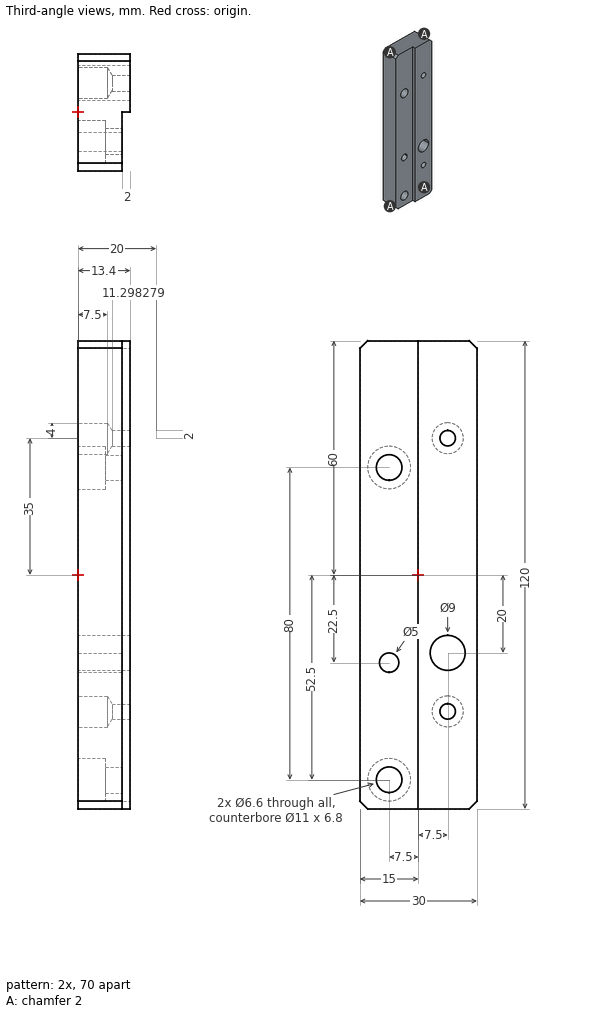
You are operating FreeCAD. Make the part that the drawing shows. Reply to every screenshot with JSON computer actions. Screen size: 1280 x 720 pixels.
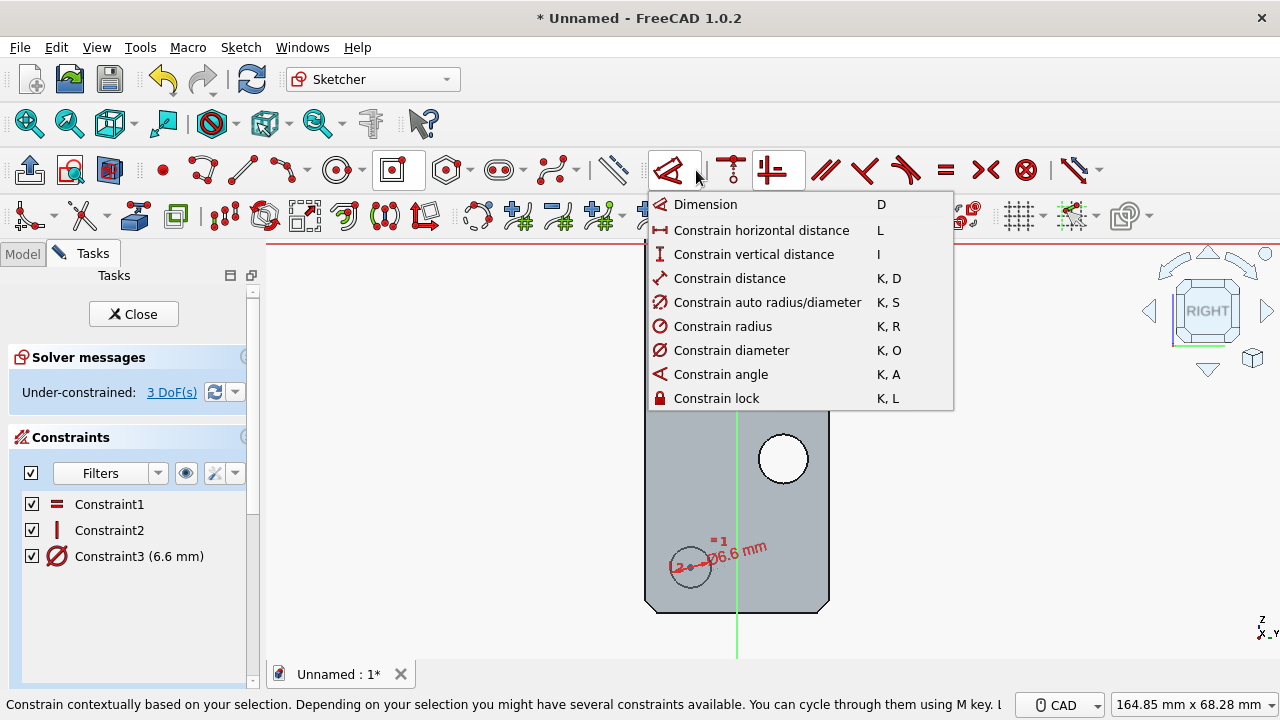
{"action": "left_click", "coordinate": [801, 230]}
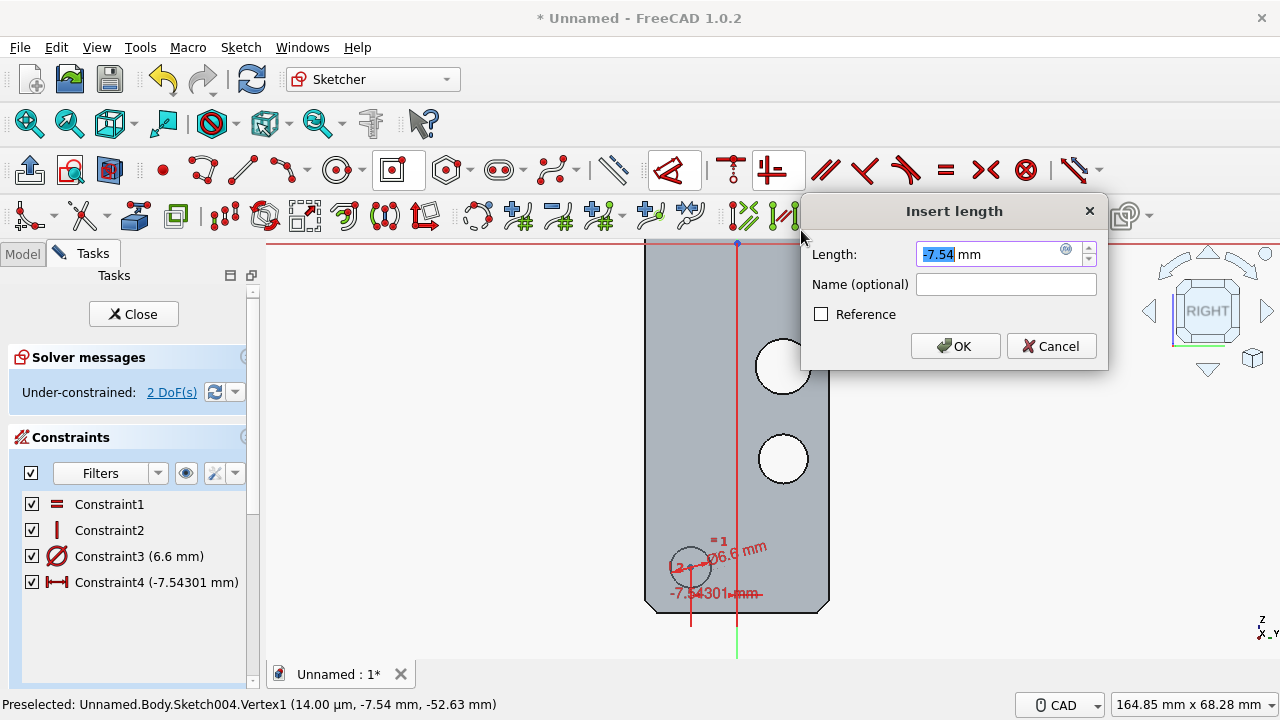
{"action": "type", "text": "-7.5"}
{"action": "key", "text": "Return"}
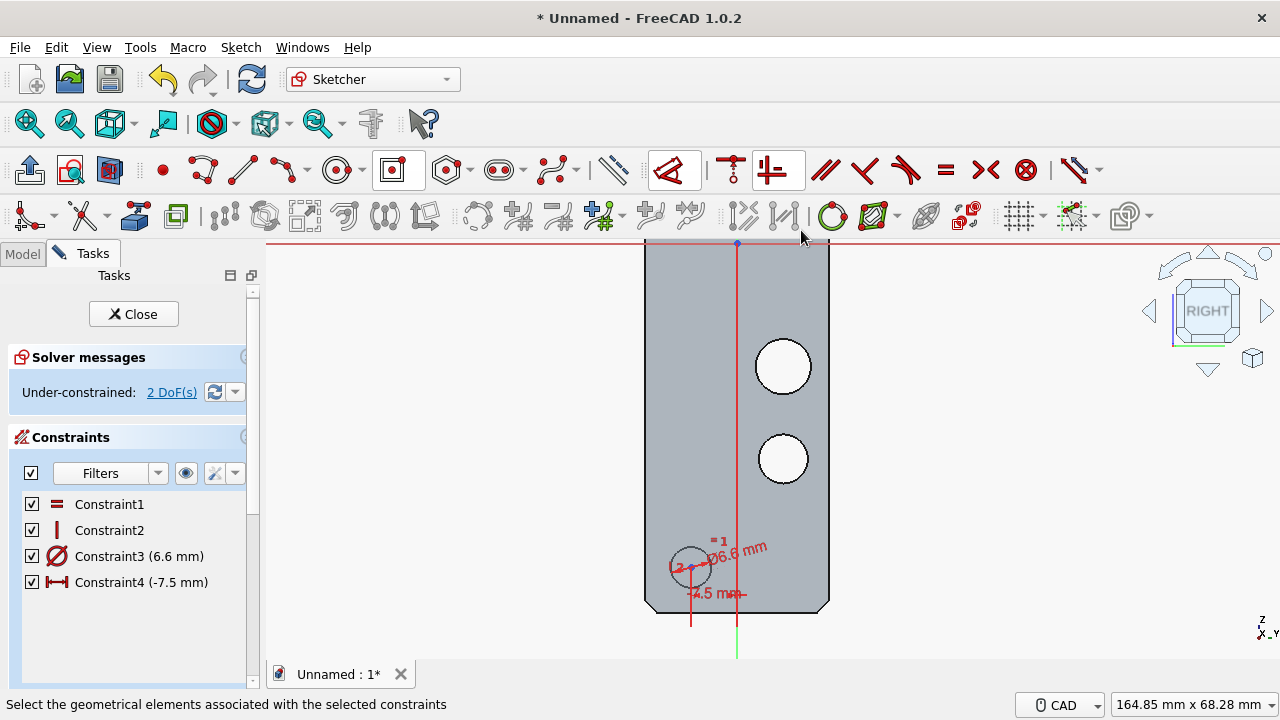
{"action": "left_click", "coordinate": [691, 567]}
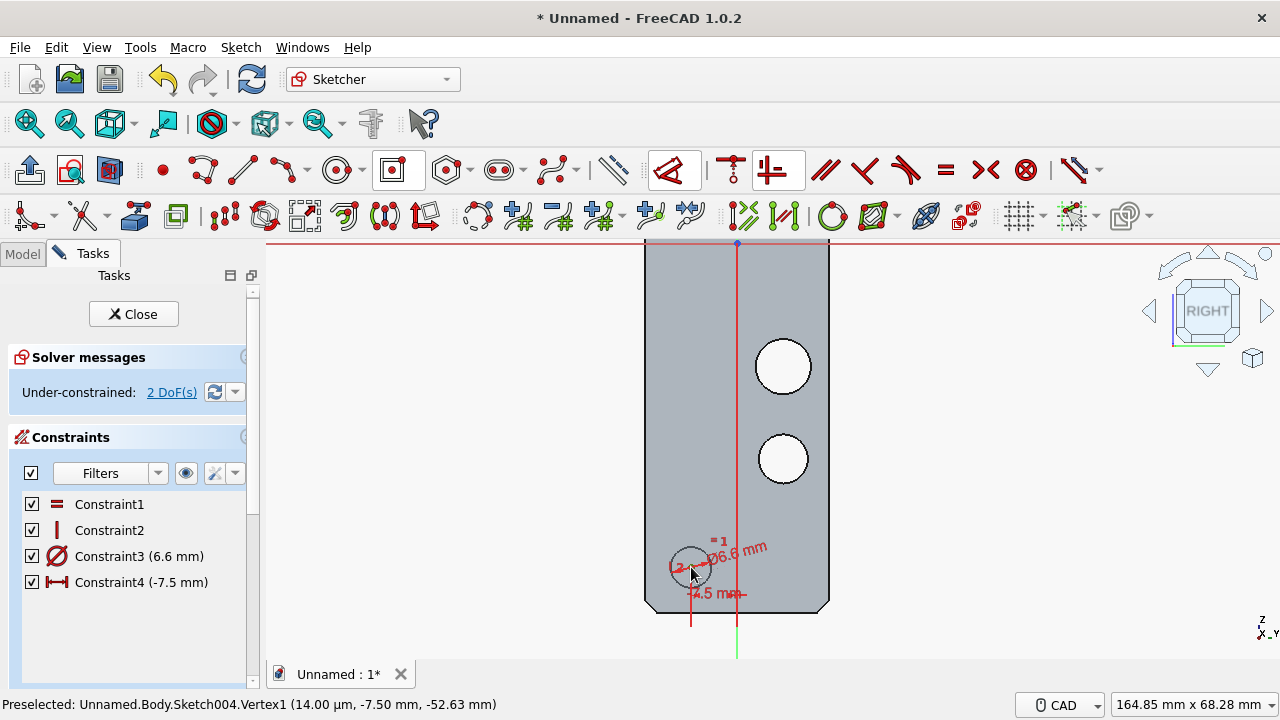
{"action": "scroll", "coordinate": [705, 554], "scroll_direction": "down", "scroll_amount": 4}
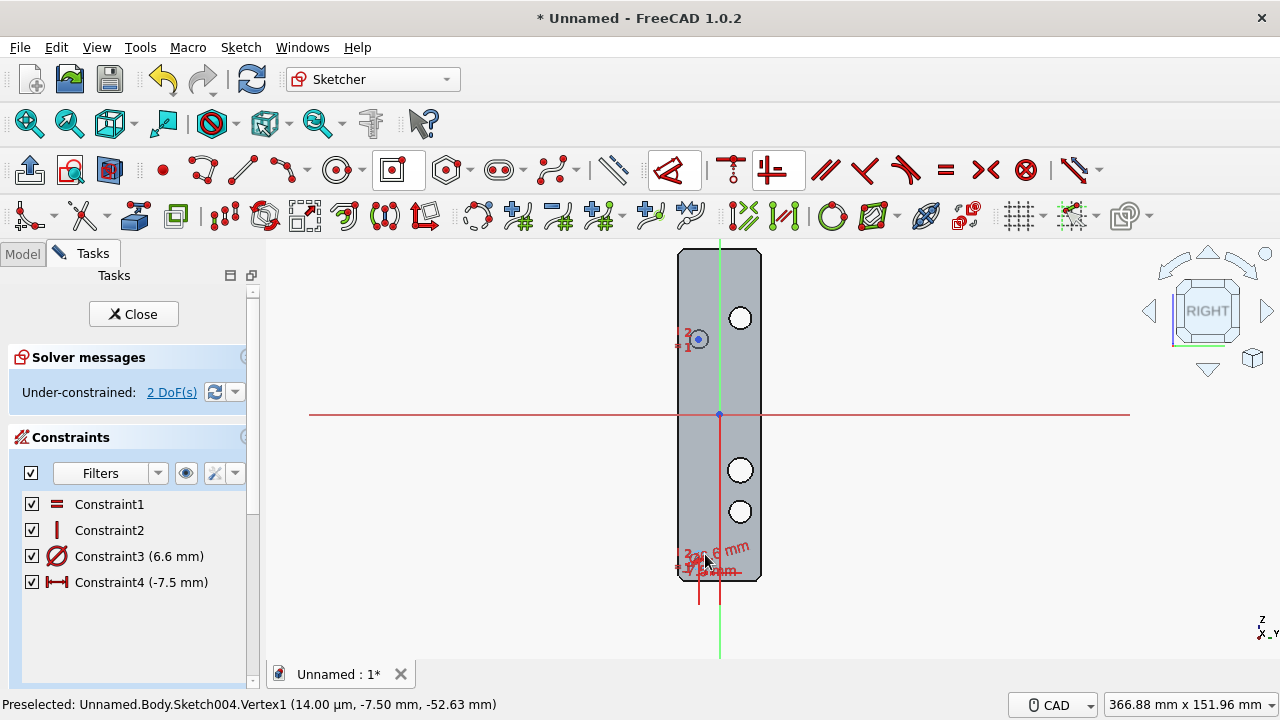
{"action": "left_click", "coordinate": [699, 339]}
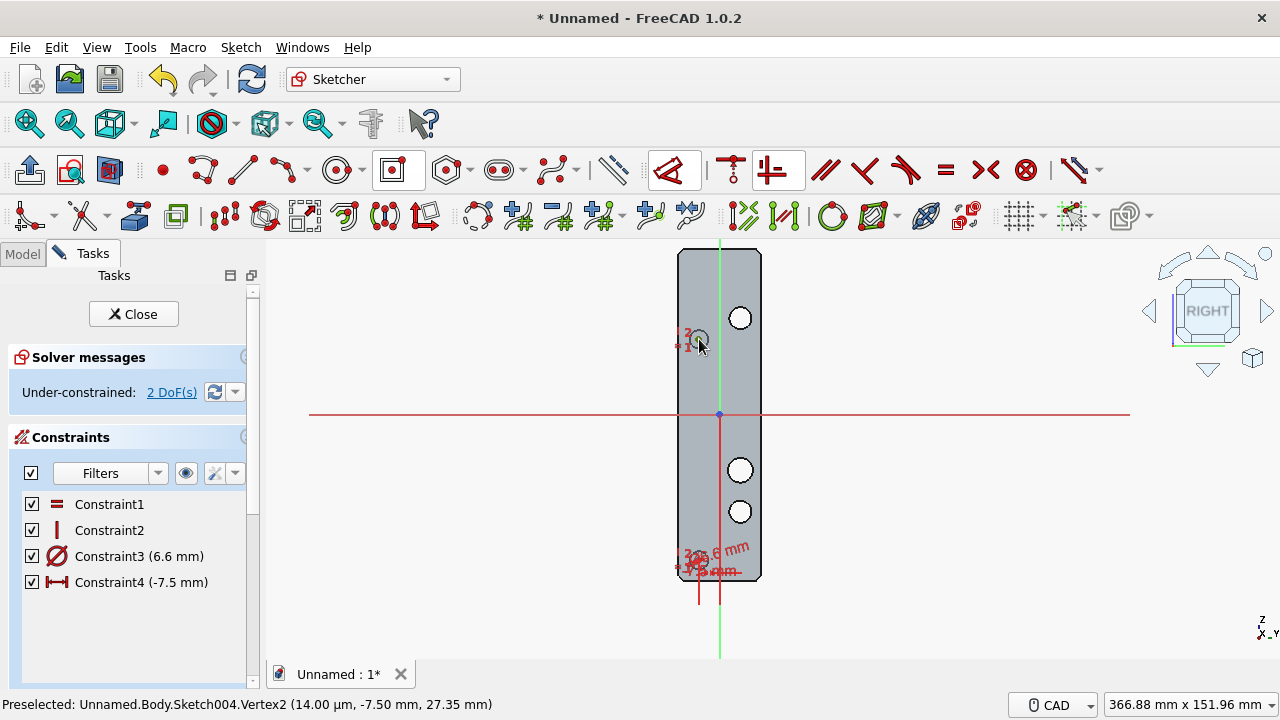
{"action": "key", "text": "i"}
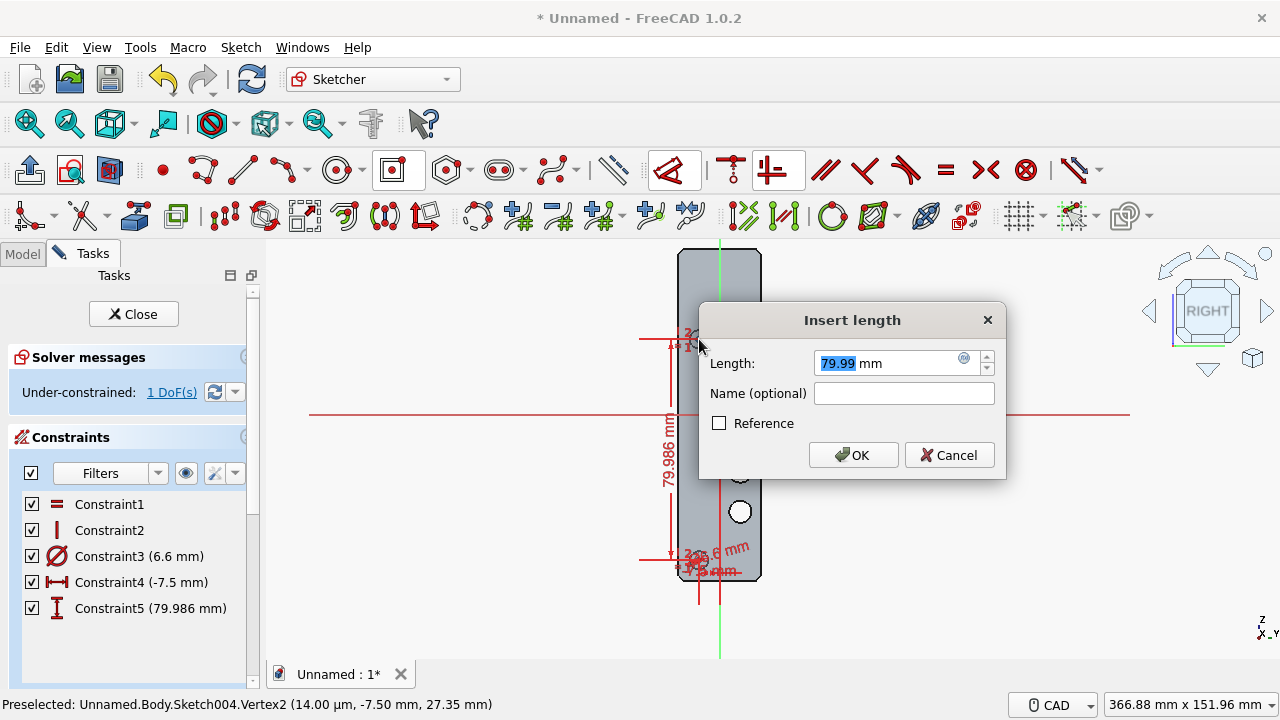
{"action": "type", "text": "80"}
{"action": "key", "text": "Return"}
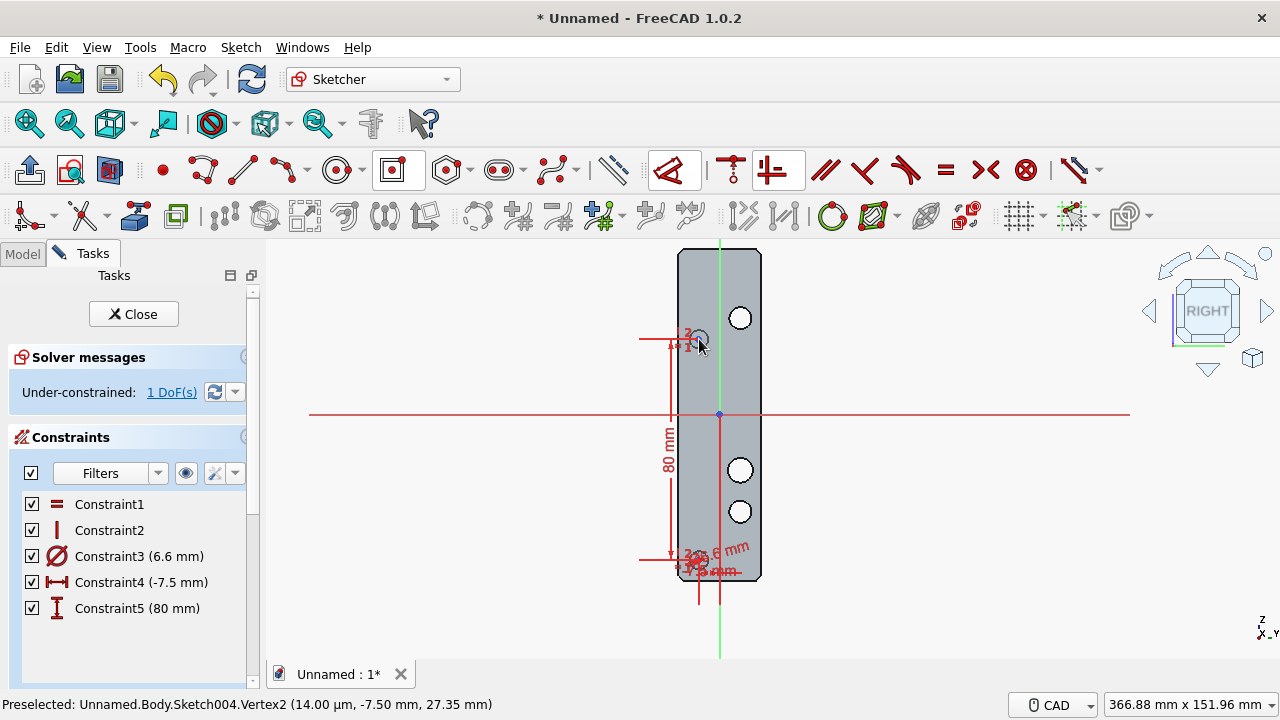
{"action": "left_click", "coordinate": [699, 560]}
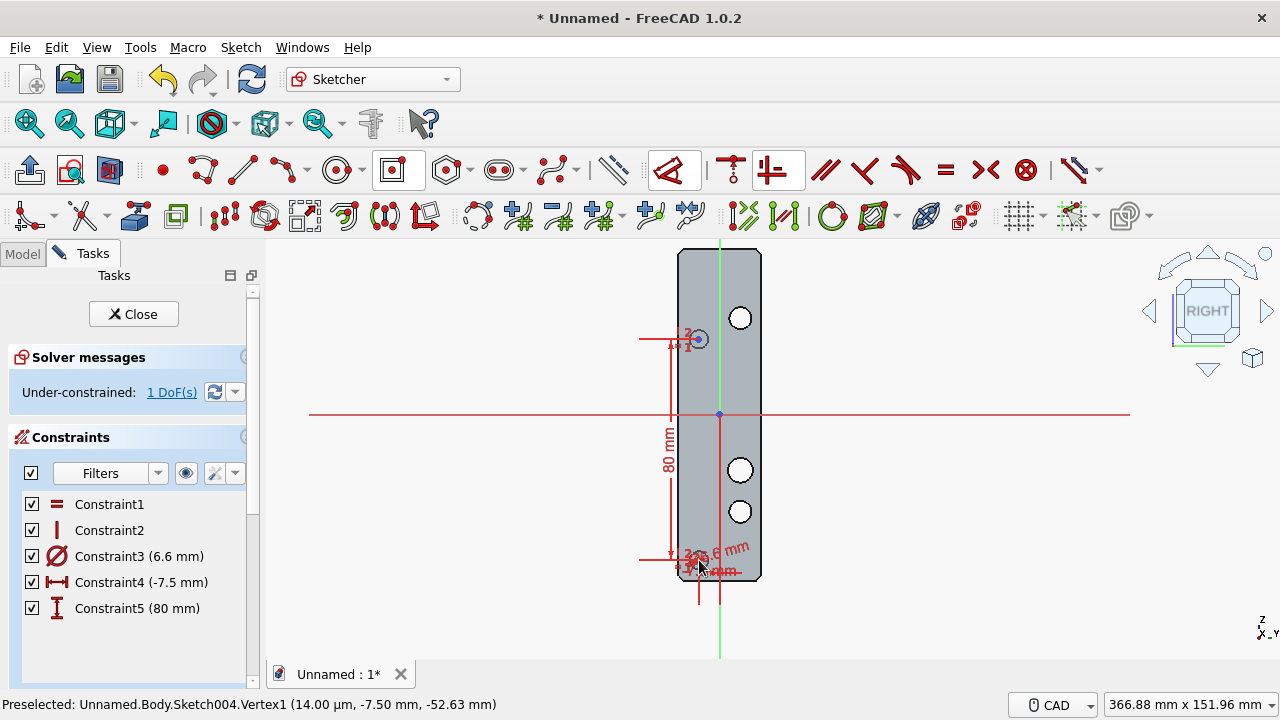
{"action": "left_click", "coordinate": [696, 170]}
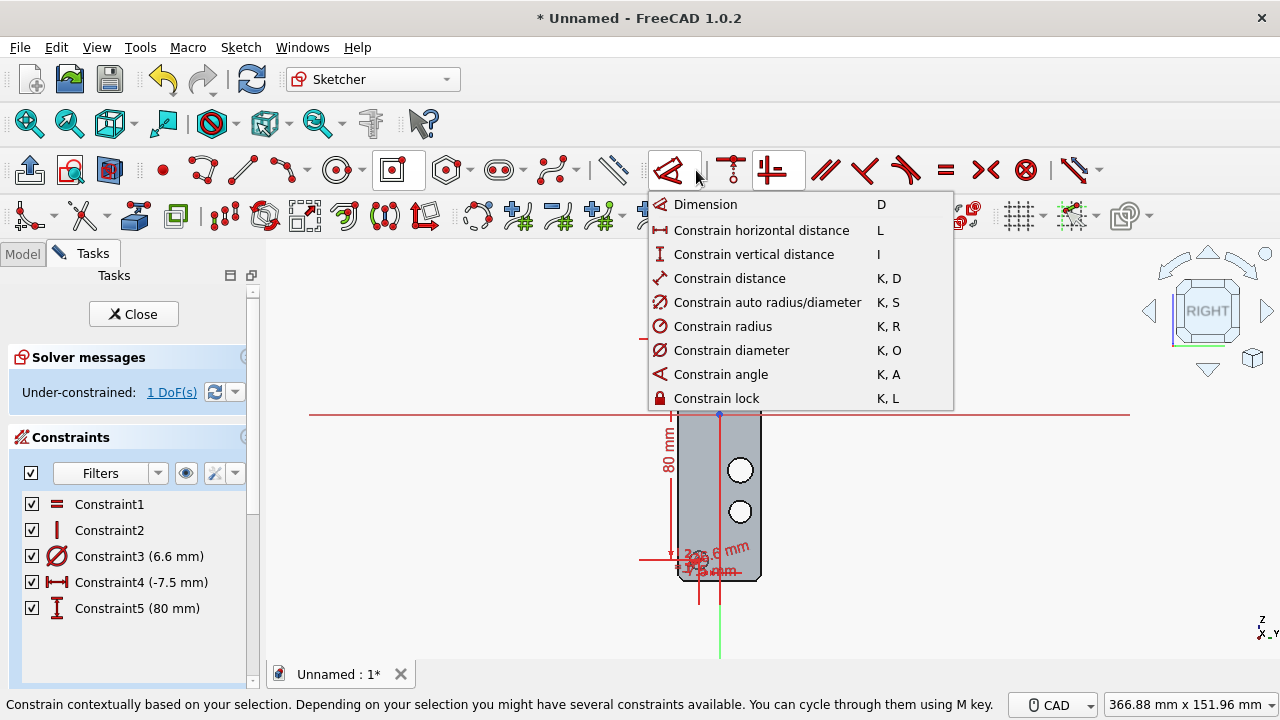
{"action": "left_click", "coordinate": [801, 254]}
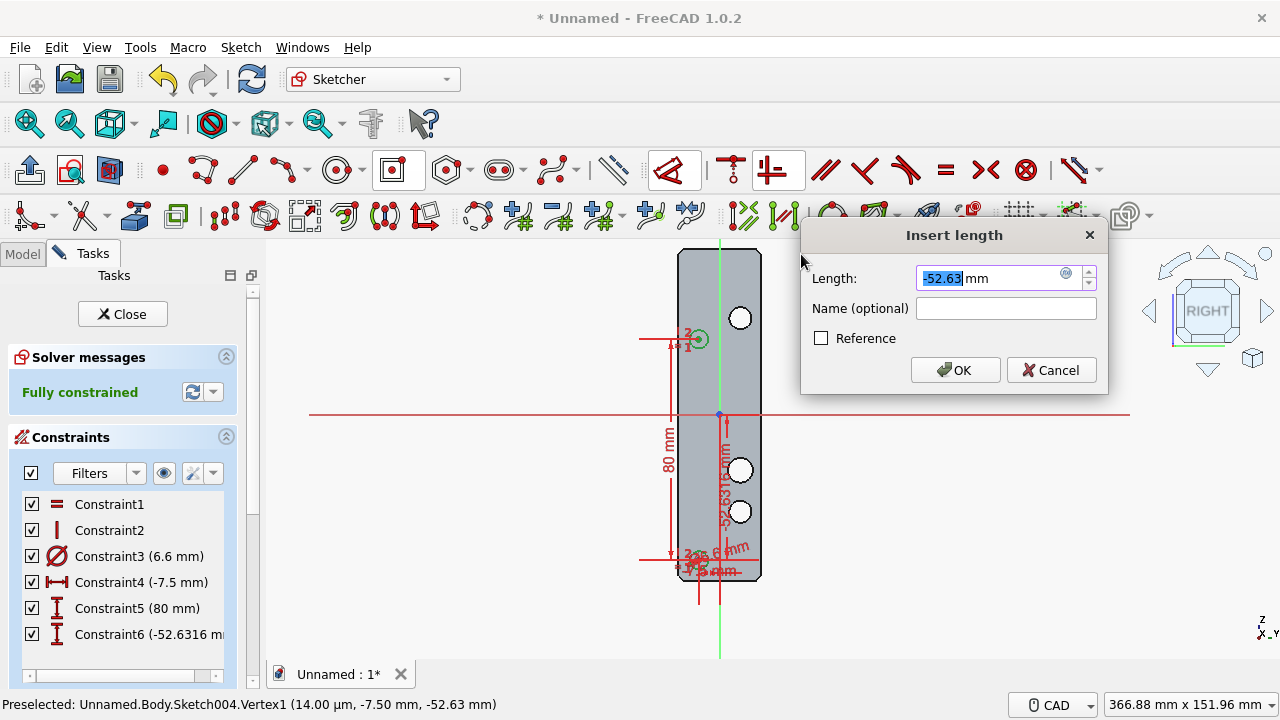
{"action": "type", "text": "-52.5"}
{"action": "key", "text": "Return"}